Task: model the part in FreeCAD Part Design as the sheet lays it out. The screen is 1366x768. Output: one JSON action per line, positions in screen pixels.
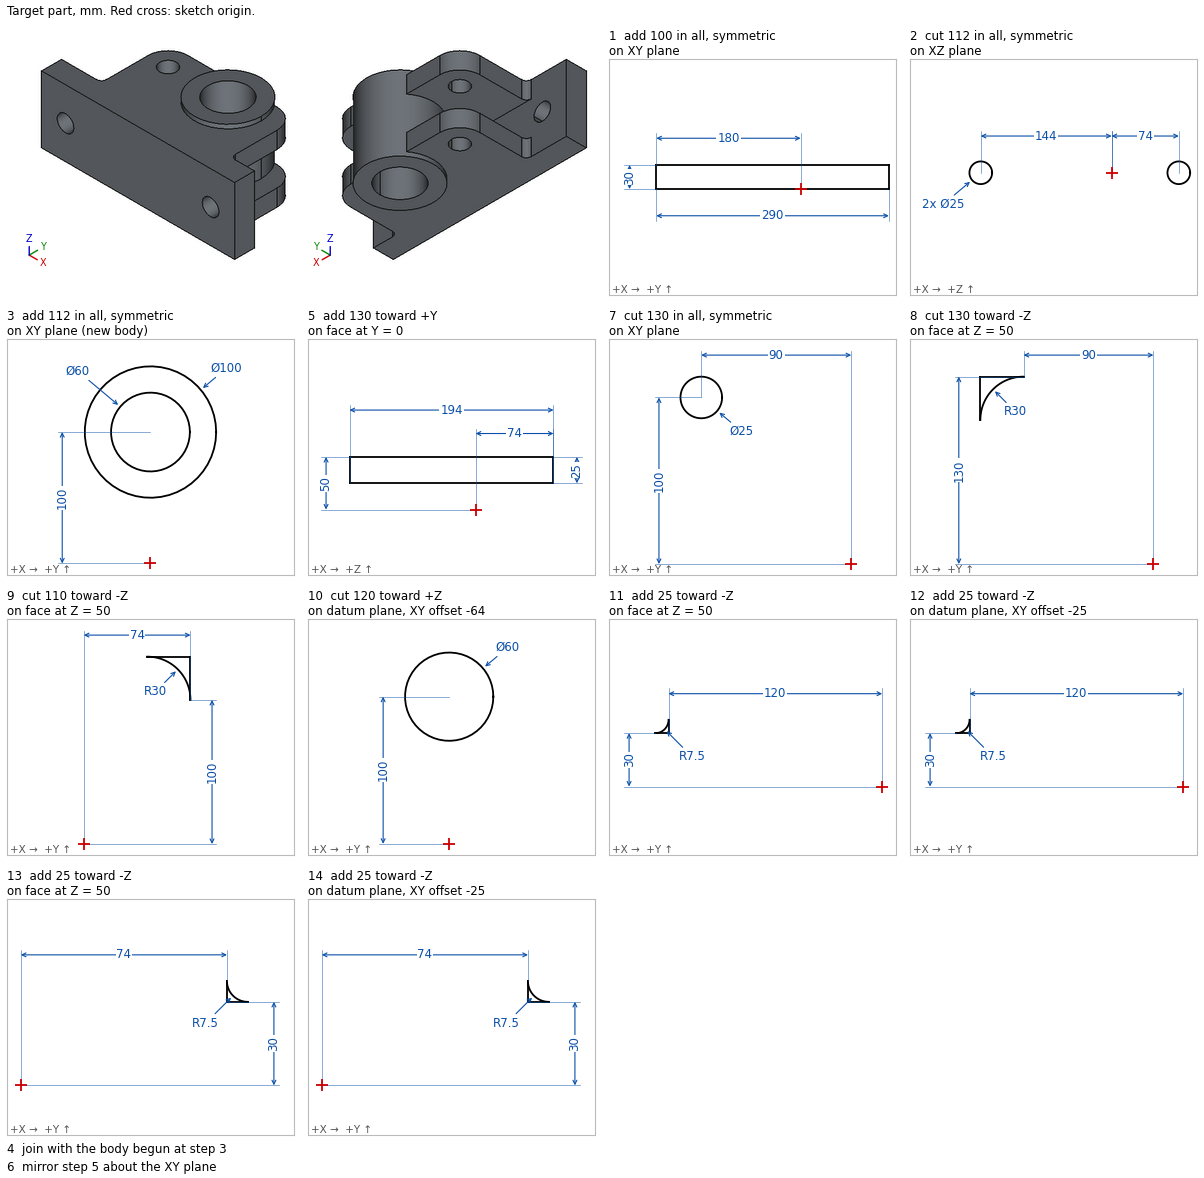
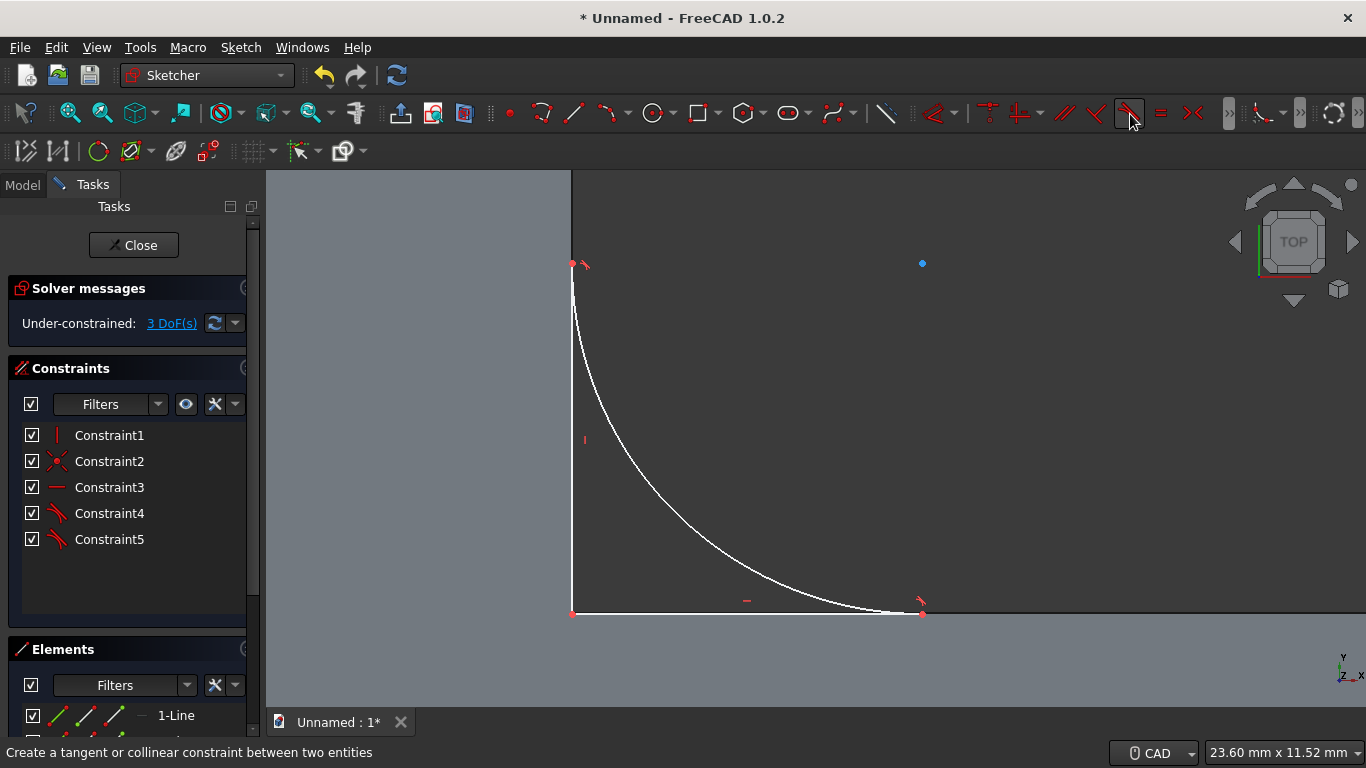
{"action": "left_click", "coordinate": [934, 114]}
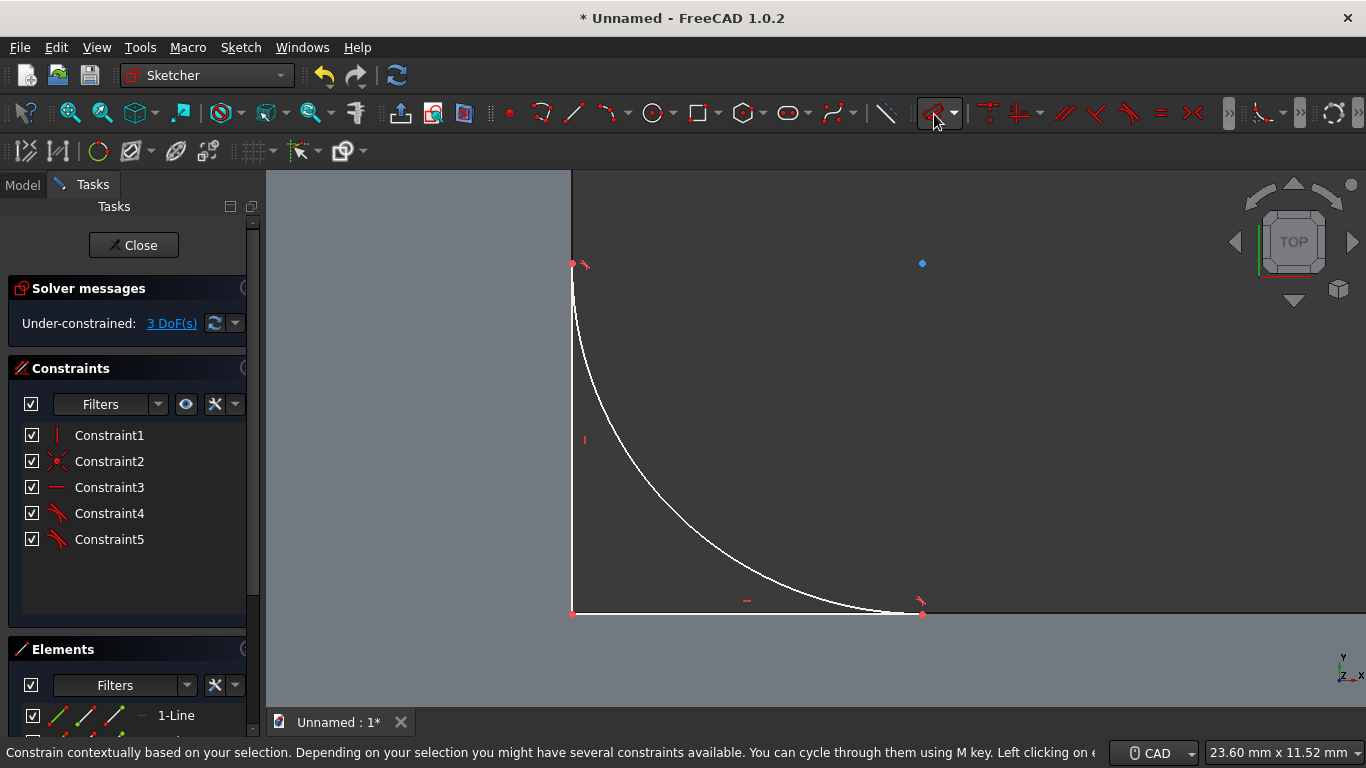
{"action": "left_click", "coordinate": [610, 423]}
{"action": "left_click", "coordinate": [540, 253]}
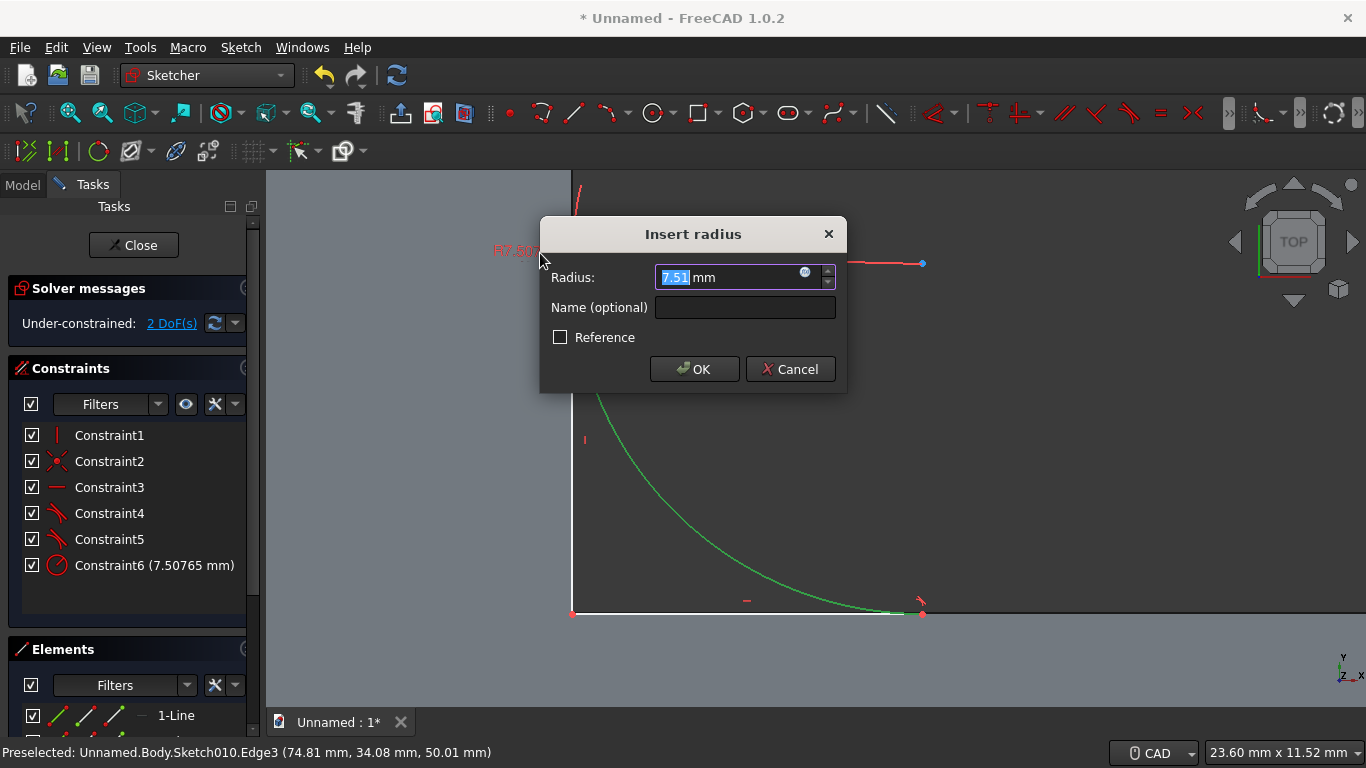
{"action": "type", "text": "7.5"}
{"action": "key", "text": "Return"}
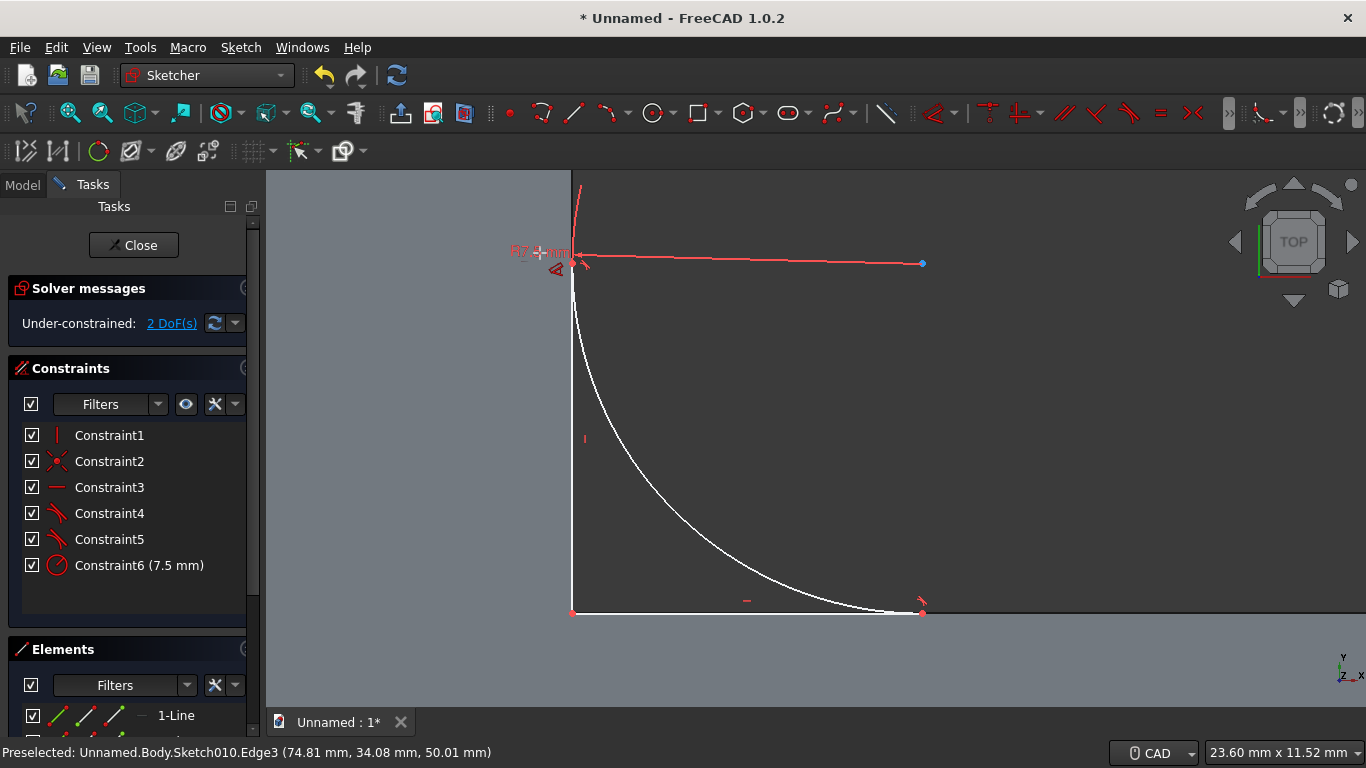
{"action": "left_click", "coordinate": [572, 264]}
{"action": "left_click", "coordinate": [433, 230]}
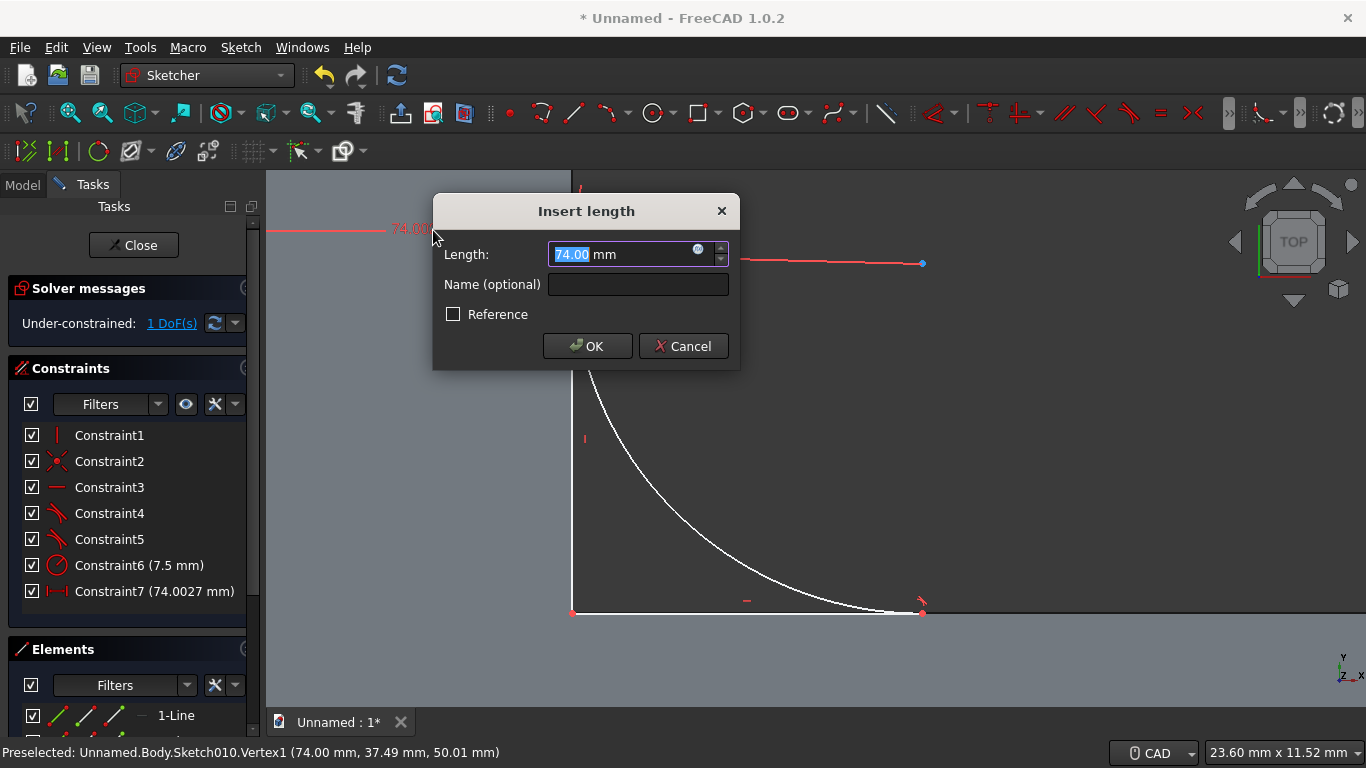
{"action": "type", "text": "74"}
{"action": "key", "text": "Return"}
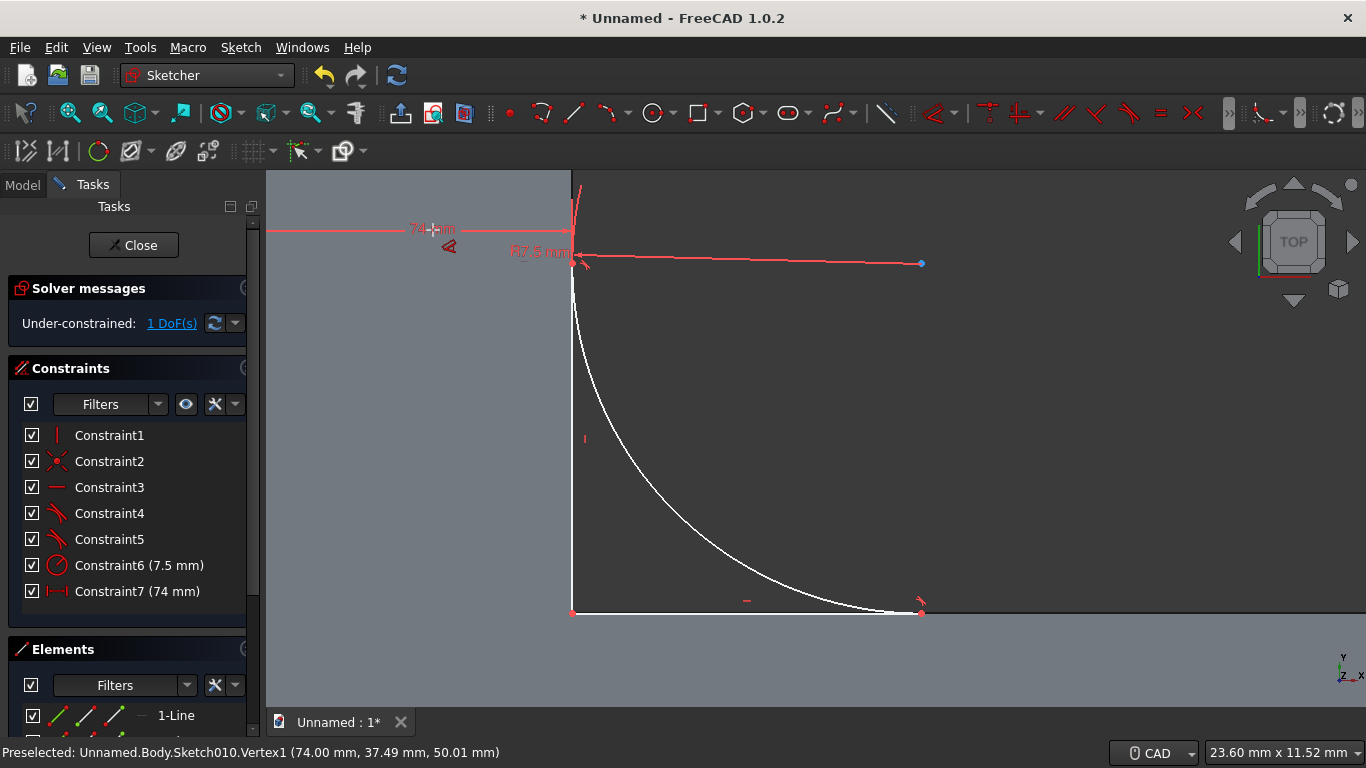
{"action": "left_click", "coordinate": [572, 614]}
{"action": "left_click", "coordinate": [606, 646]}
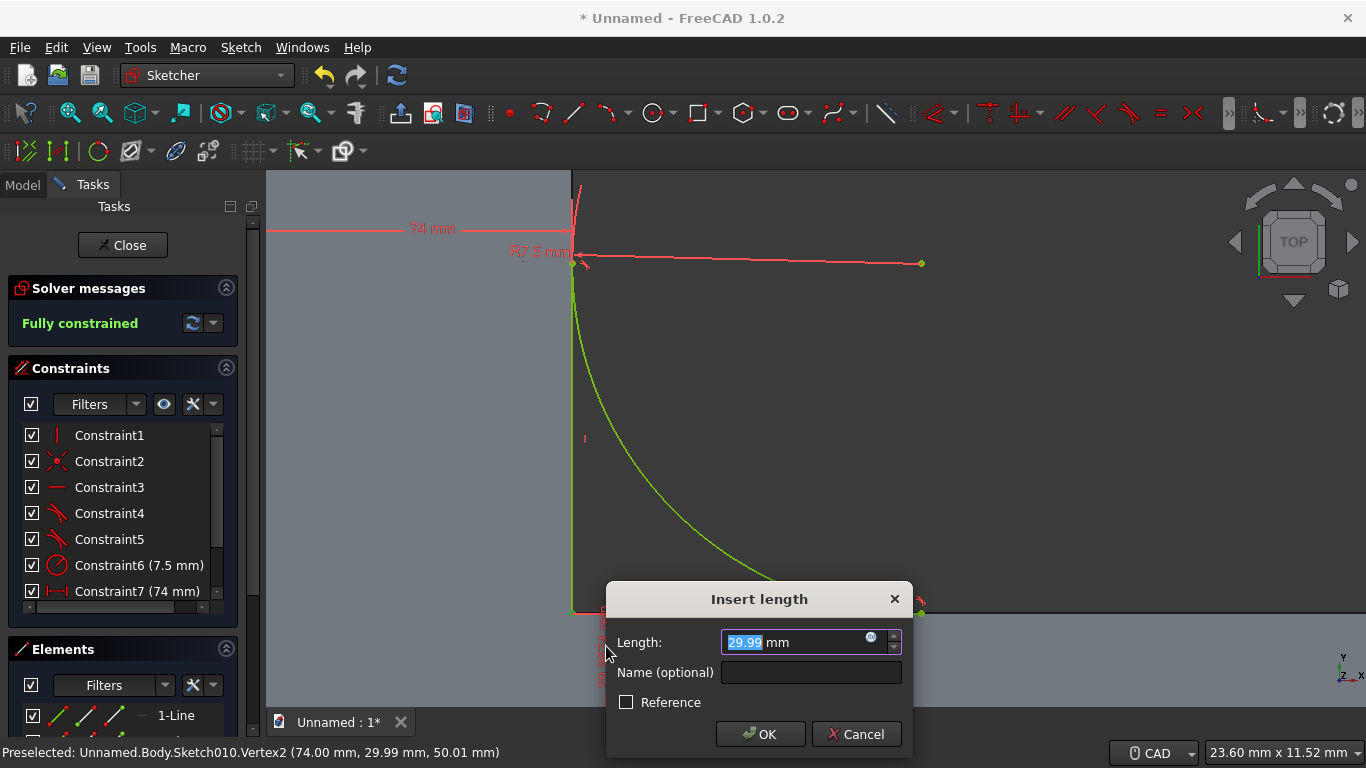
{"action": "type", "text": "30"}
{"action": "key", "text": "Return"}
{"action": "key", "text": "Escape"}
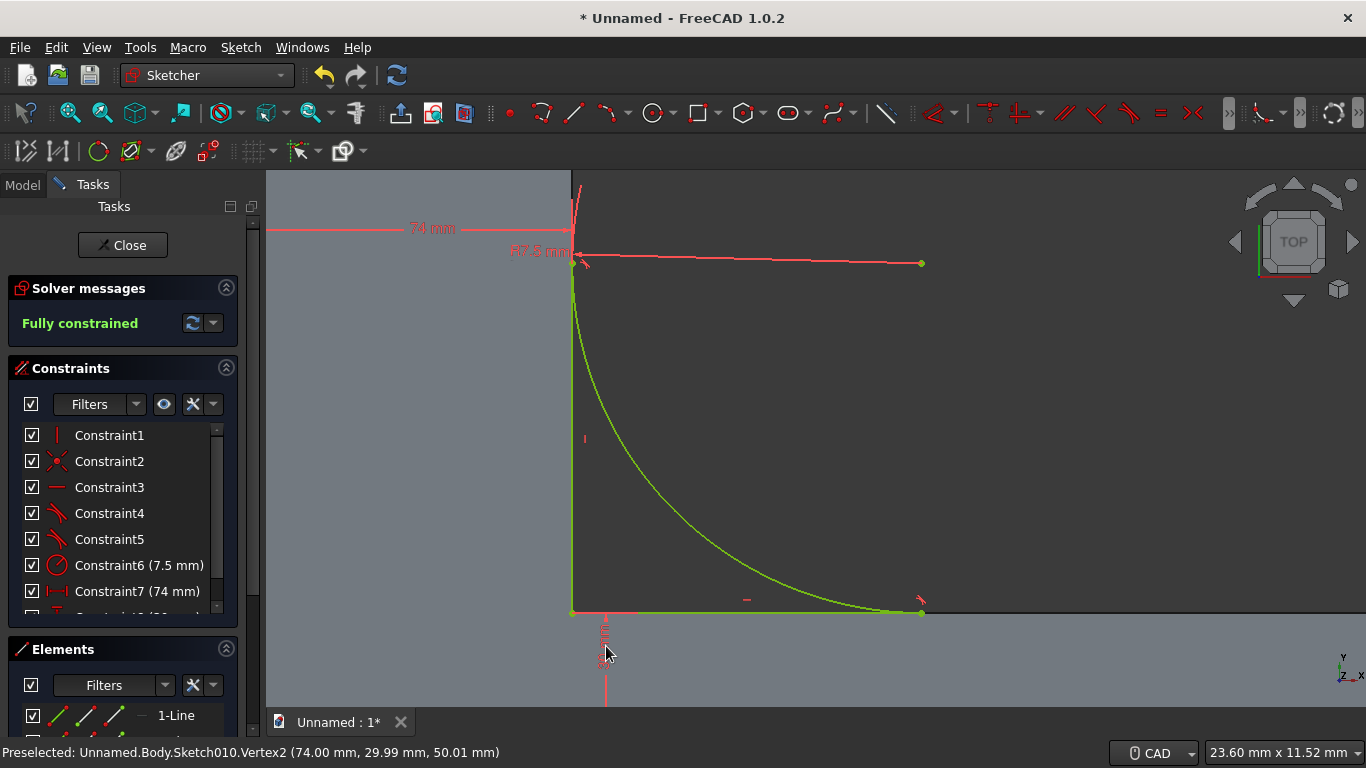
{"action": "left_click", "coordinate": [123, 245]}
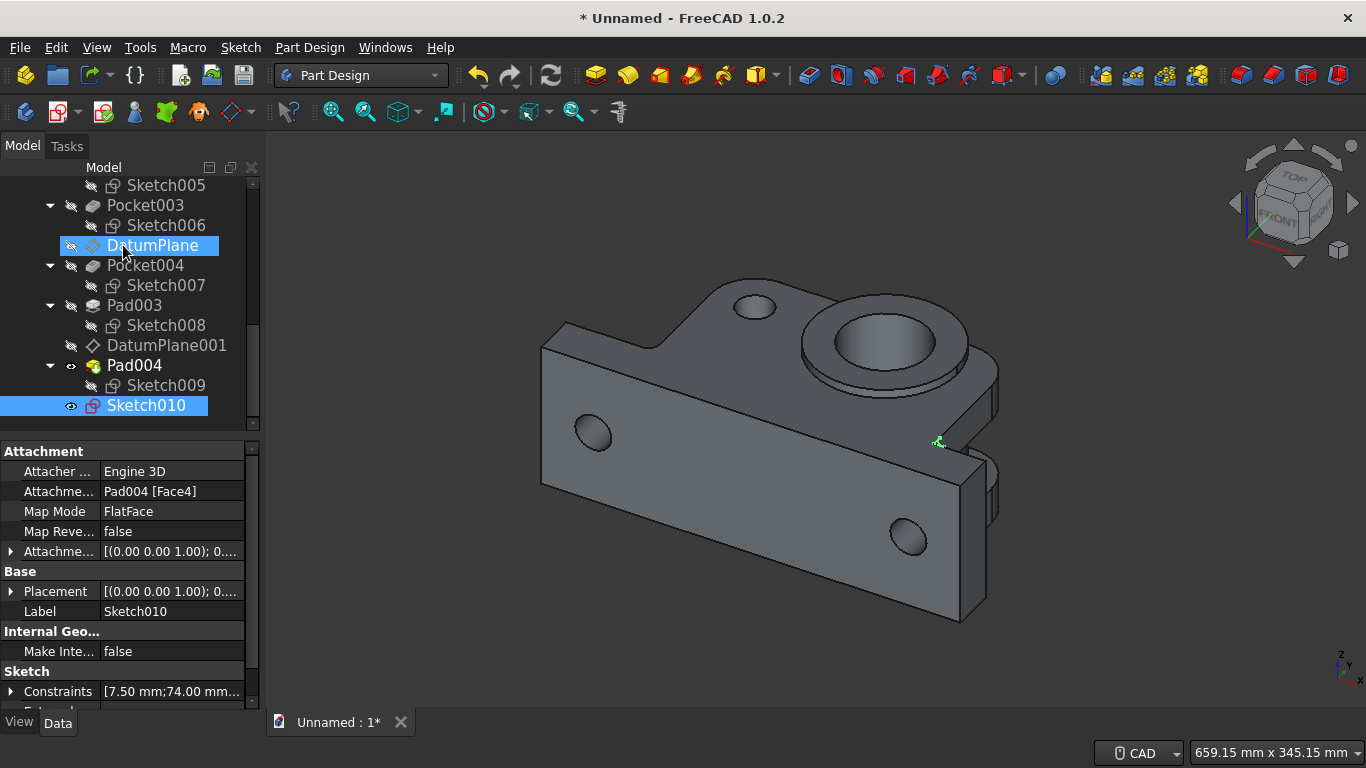
{"action": "left_click", "coordinate": [596, 76]}